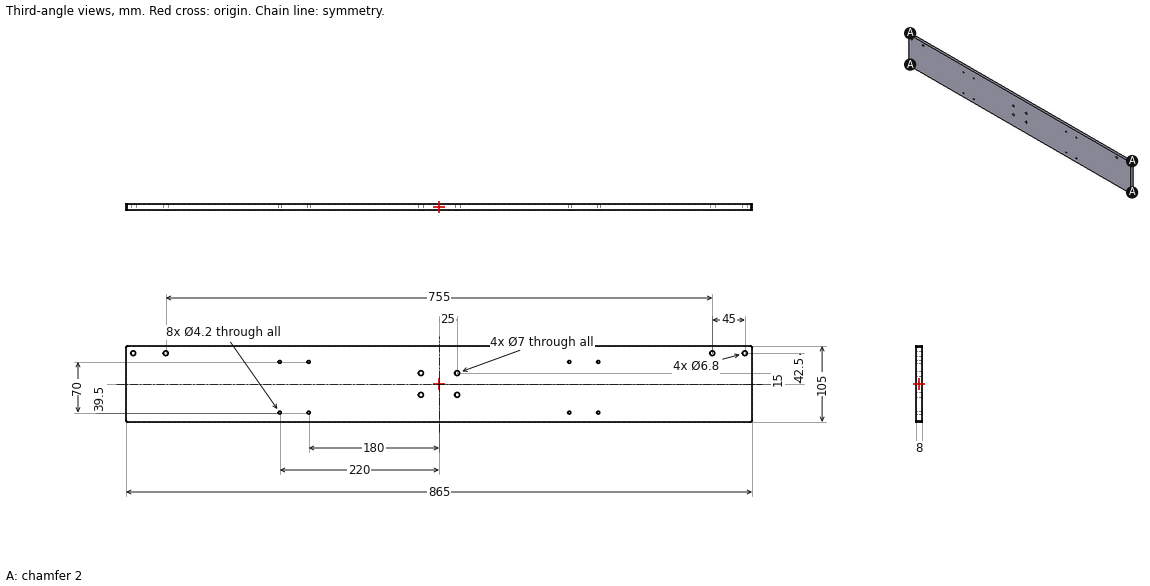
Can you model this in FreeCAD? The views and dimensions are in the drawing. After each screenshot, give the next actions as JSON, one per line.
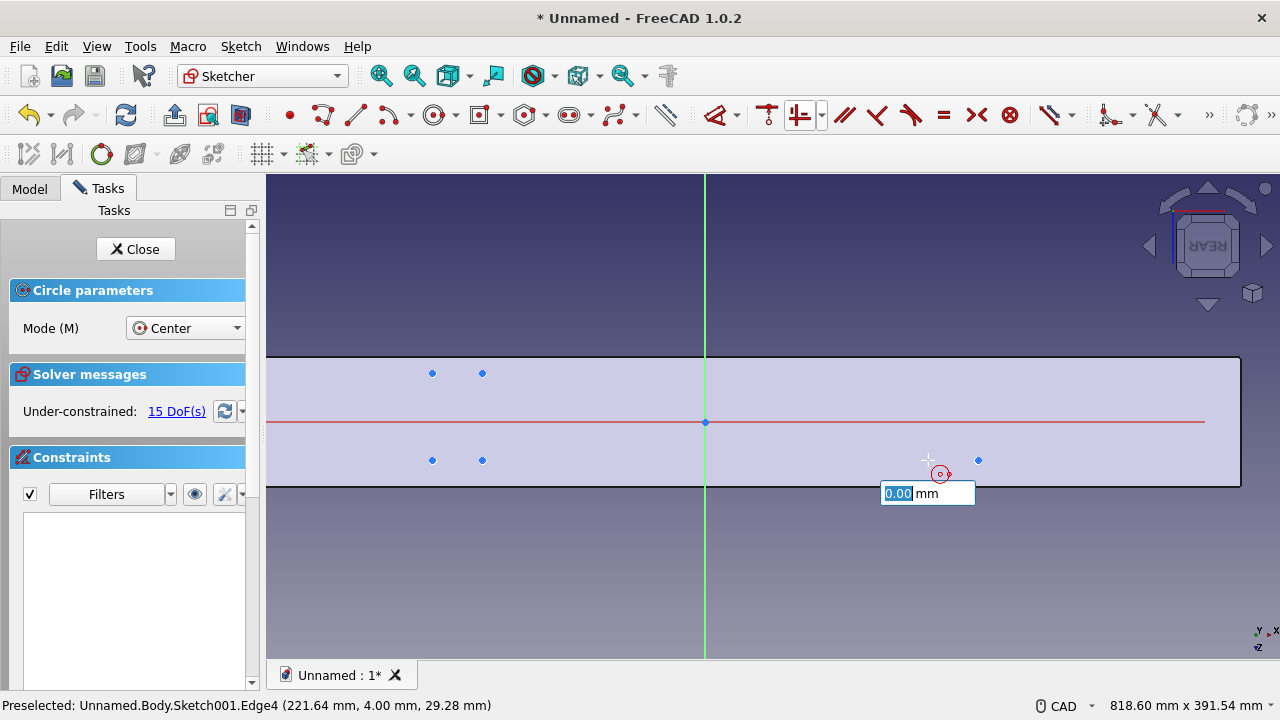
{"action": "scroll", "coordinate": [930, 458], "scroll_direction": "up", "scroll_amount": 10}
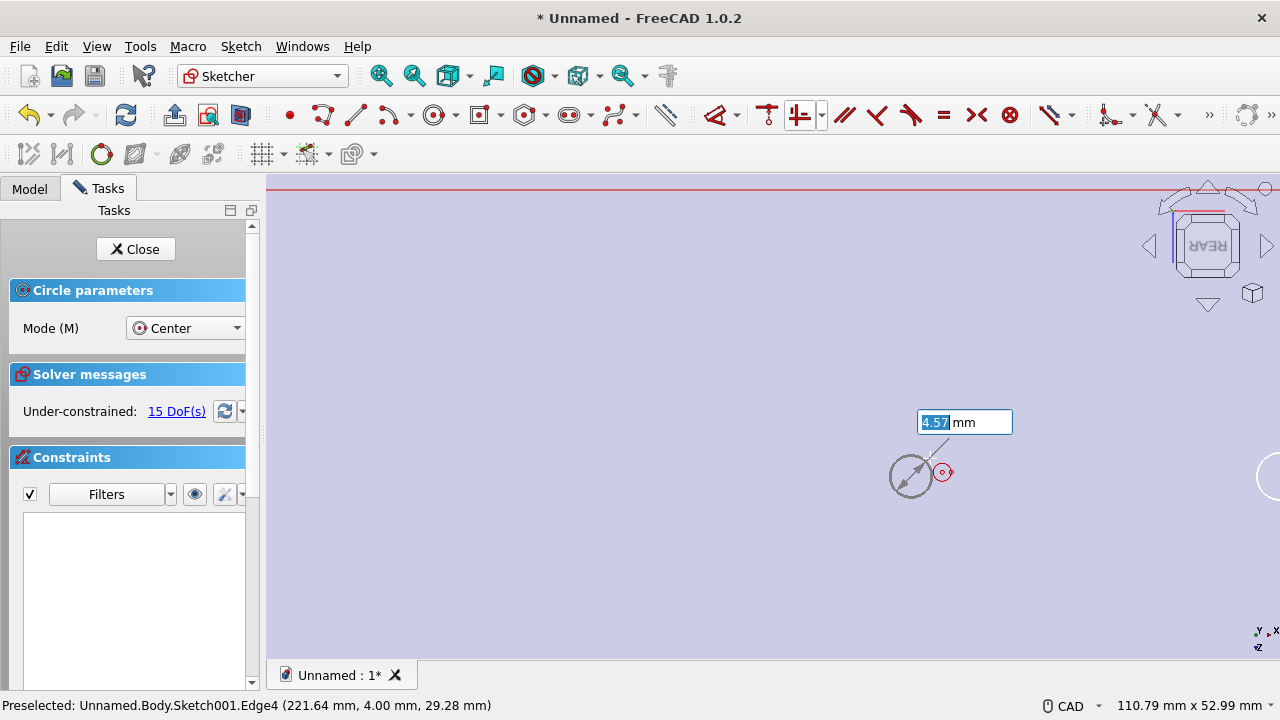
{"action": "left_click", "coordinate": [928, 456]}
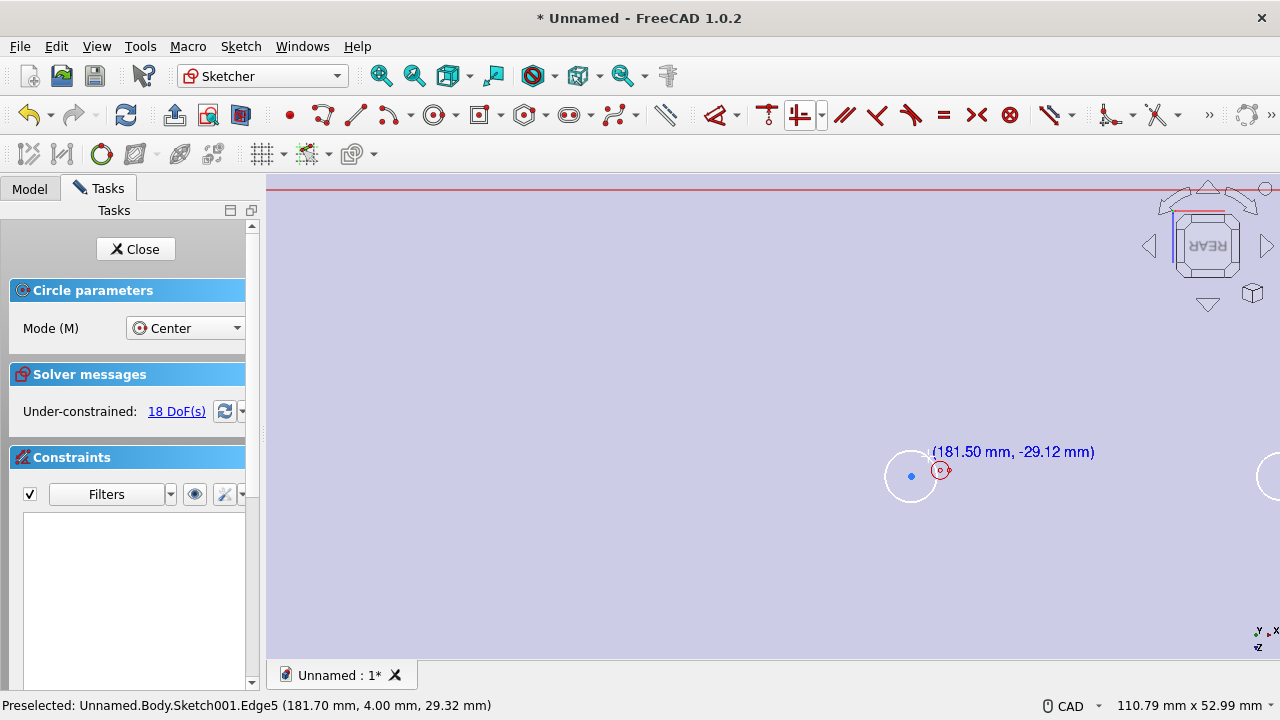
{"action": "scroll", "coordinate": [930, 458], "scroll_direction": "down", "scroll_amount": 10}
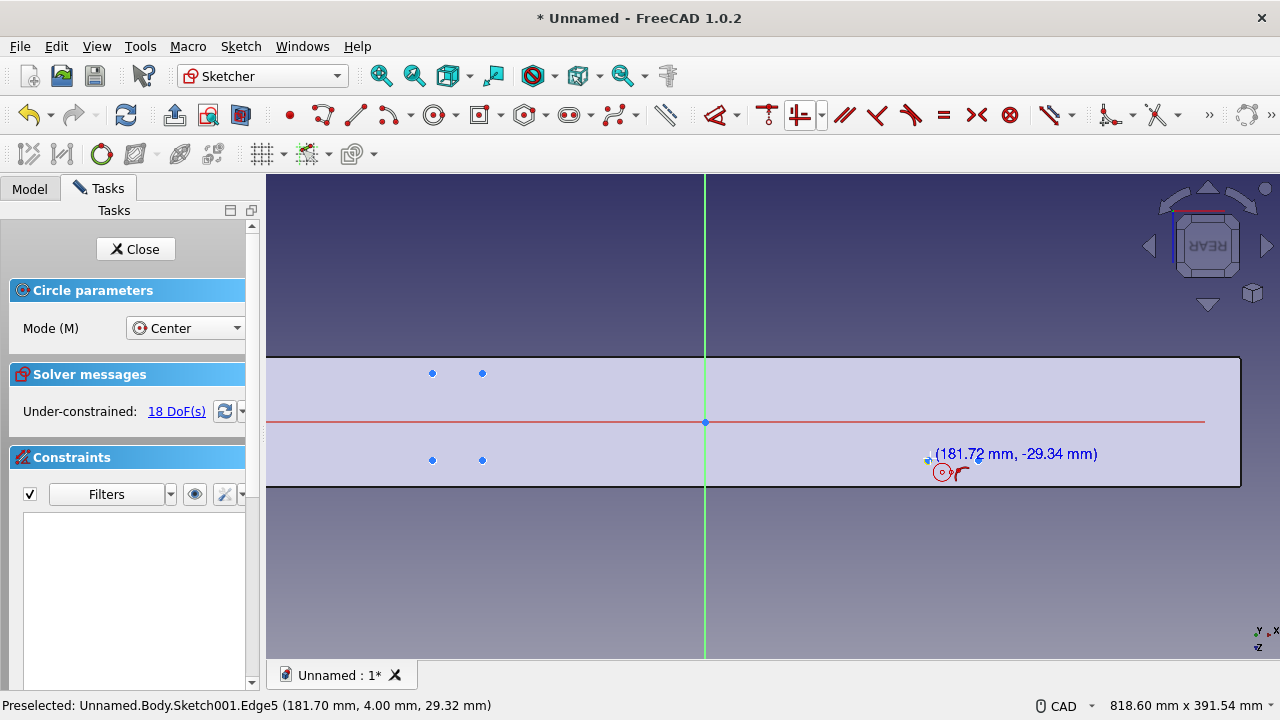
{"action": "scroll", "coordinate": [928, 373], "scroll_direction": "up", "scroll_amount": 11}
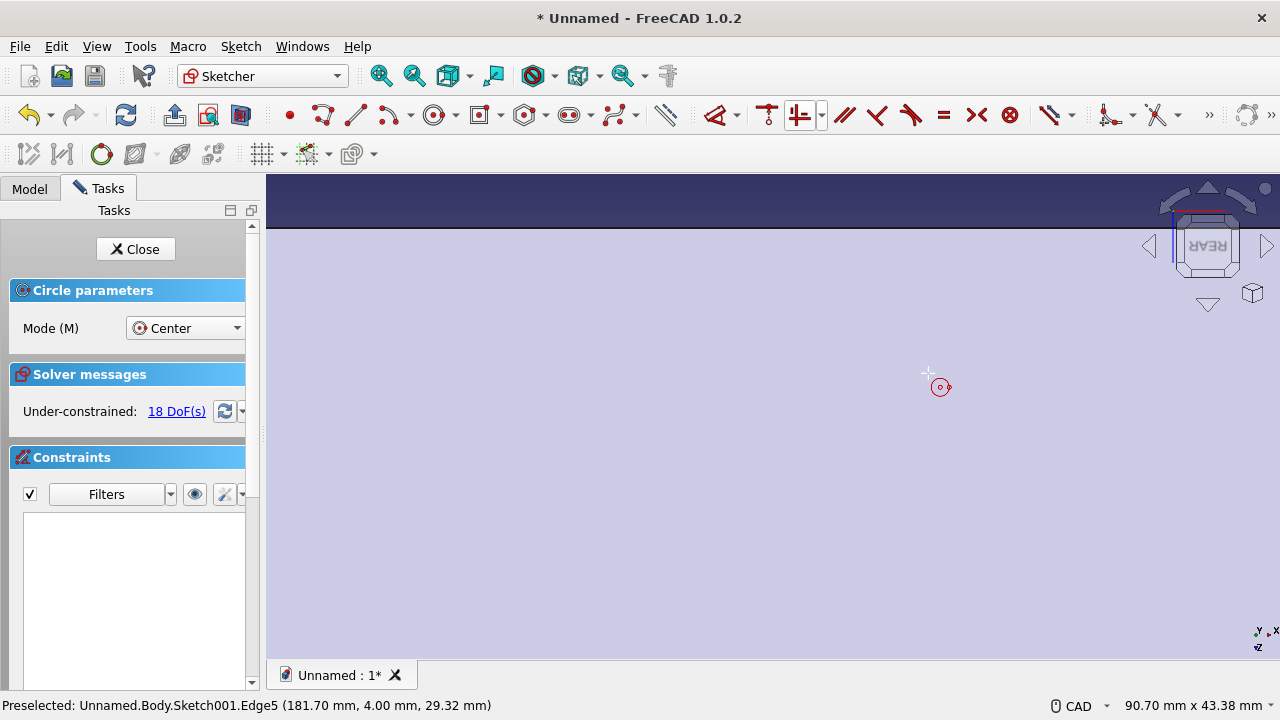
{"action": "scroll", "coordinate": [928, 373], "scroll_direction": "down", "scroll_amount": 11}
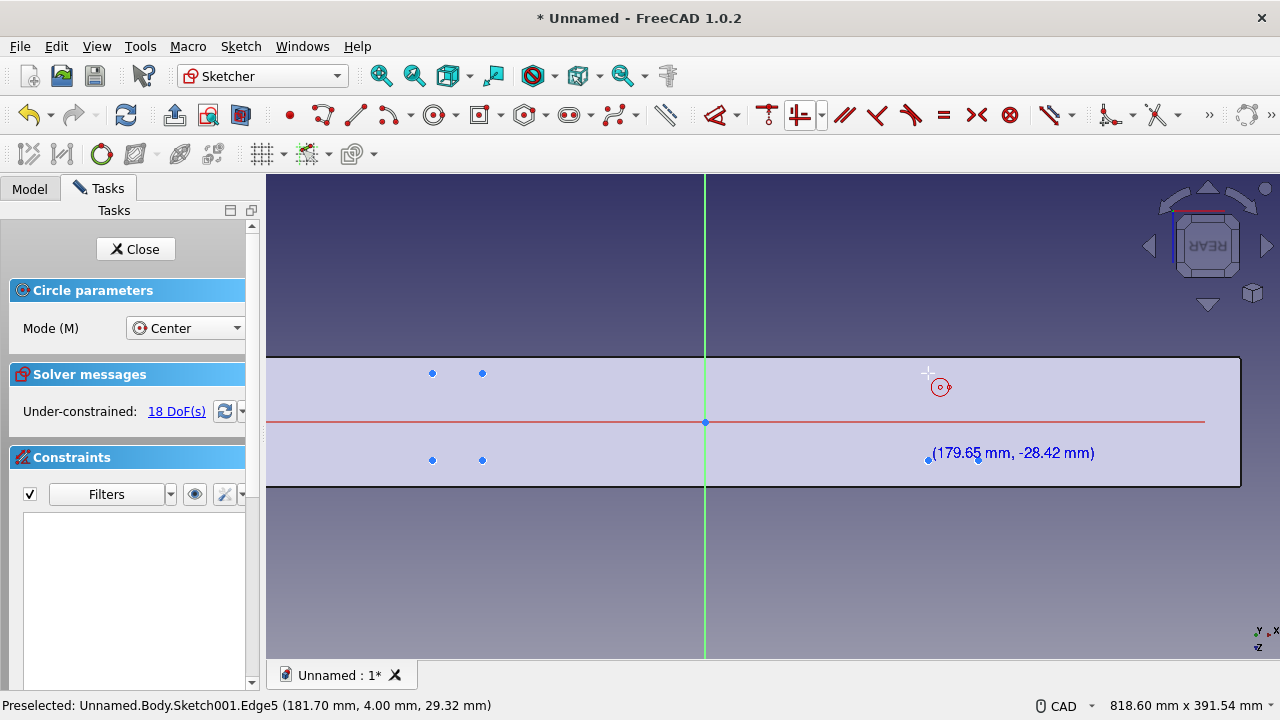
{"action": "left_click", "coordinate": [928, 373]}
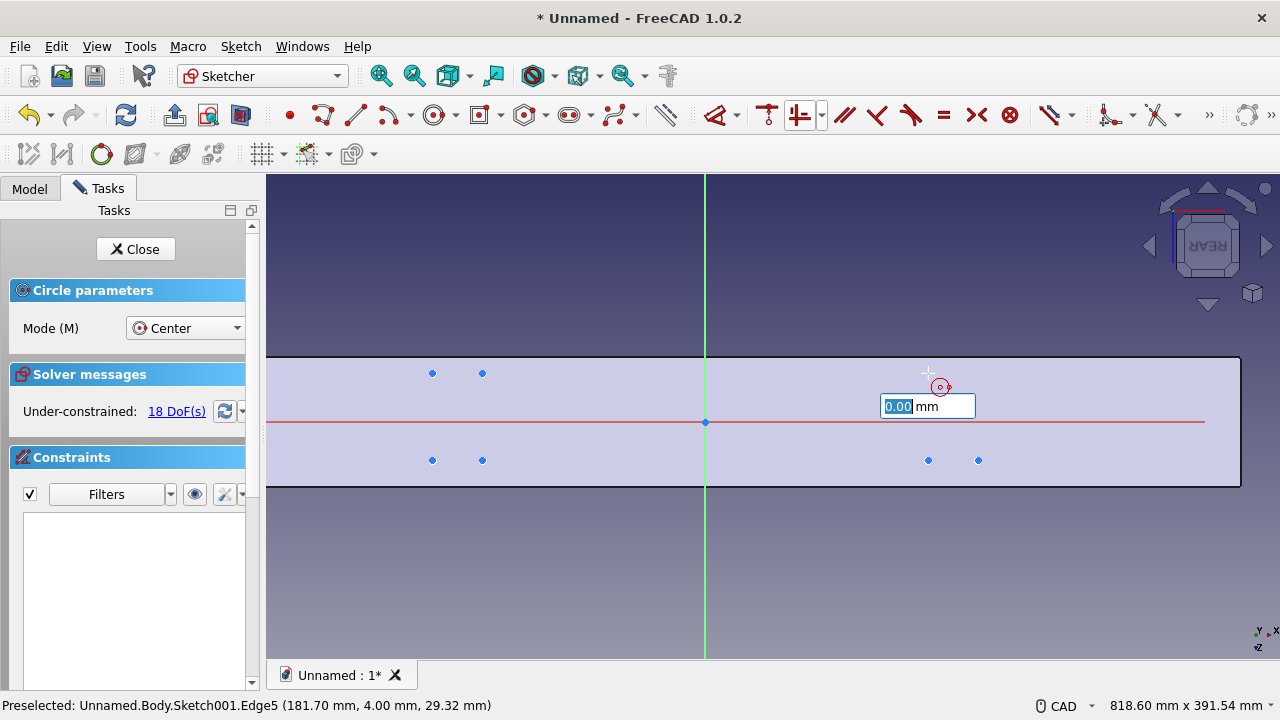
{"action": "scroll", "coordinate": [930, 372], "scroll_direction": "up", "scroll_amount": 10}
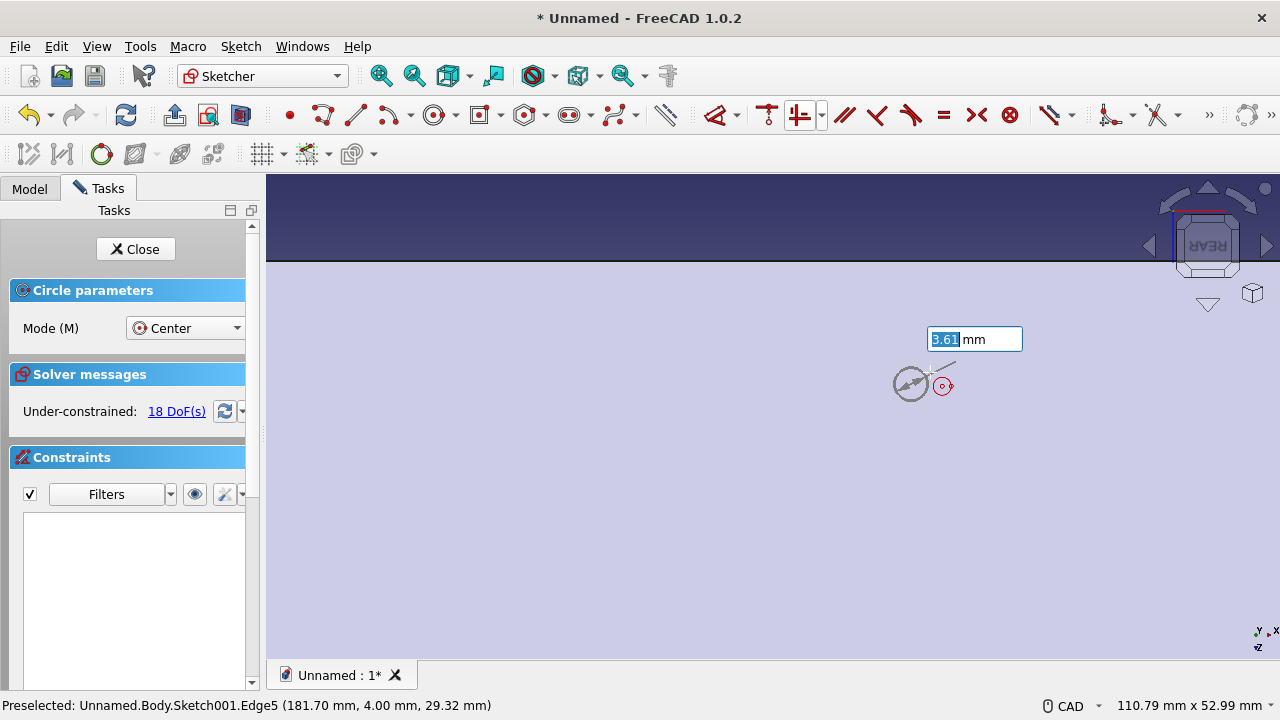
{"action": "left_click", "coordinate": [928, 366]}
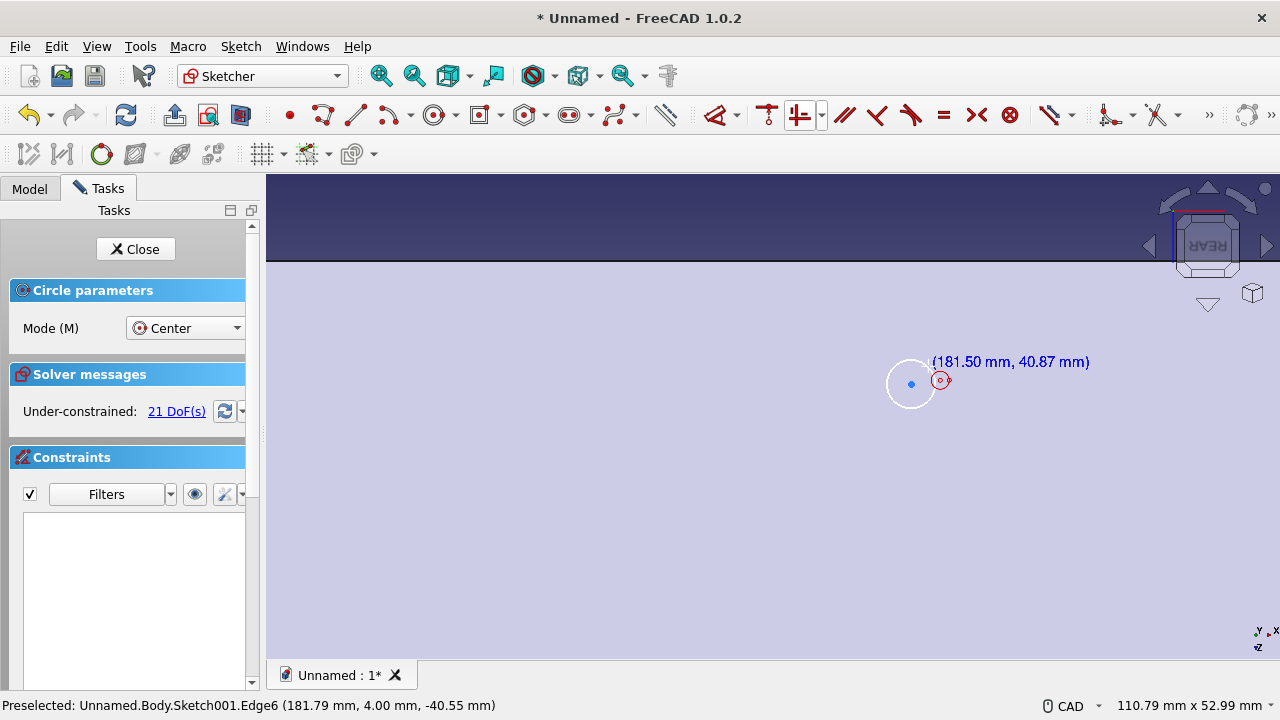
{"action": "scroll", "coordinate": [930, 372], "scroll_direction": "down", "scroll_amount": 10}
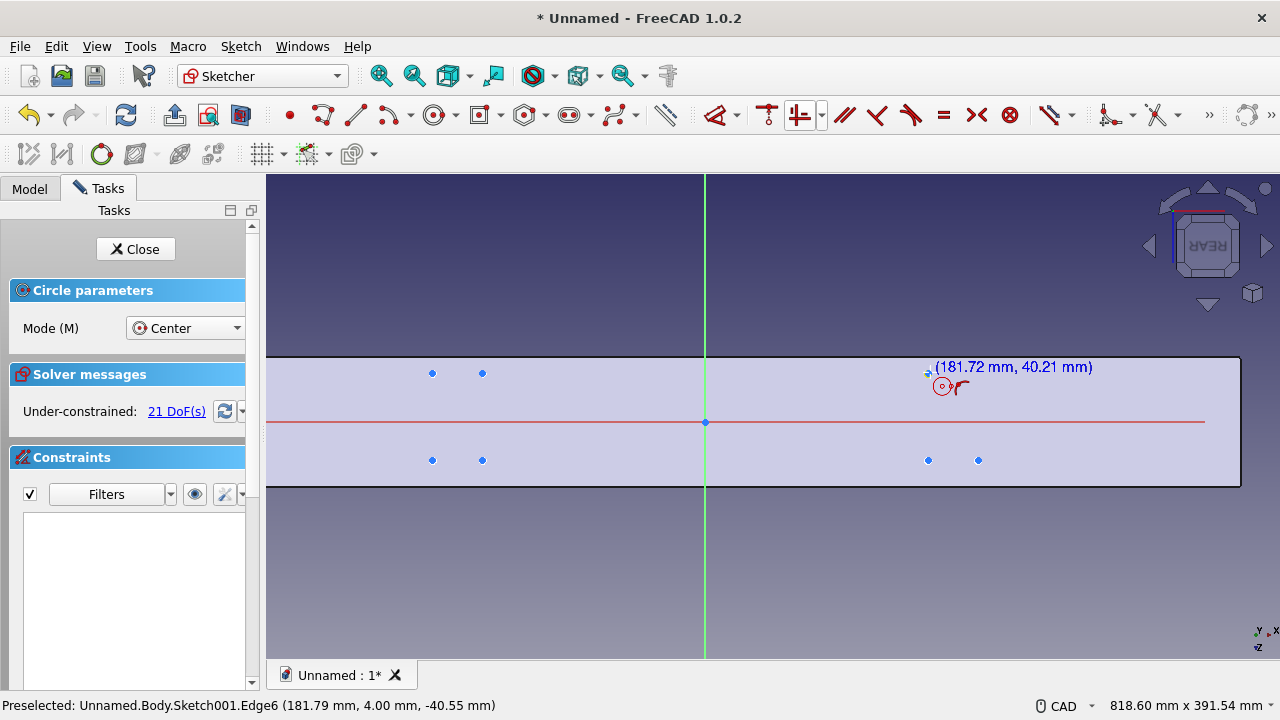
{"action": "scroll", "coordinate": [978, 373], "scroll_direction": "up", "scroll_amount": 11}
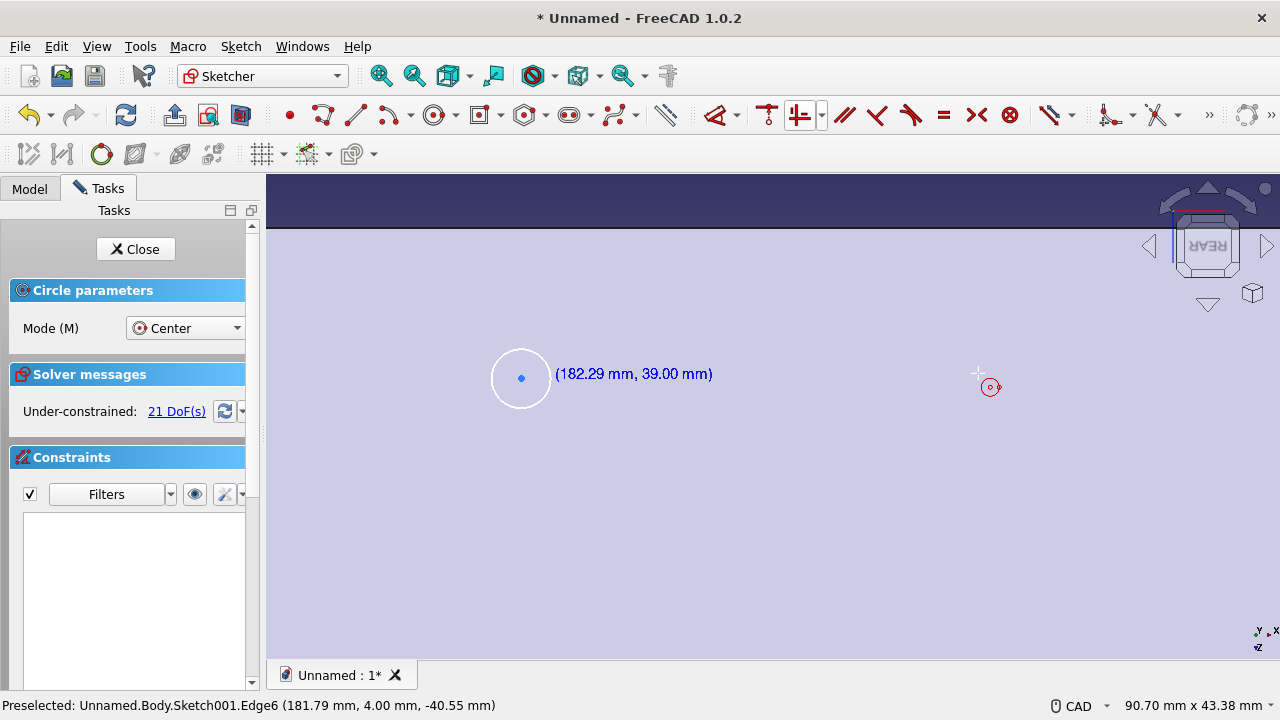
{"action": "scroll", "coordinate": [978, 373], "scroll_direction": "down", "scroll_amount": 11}